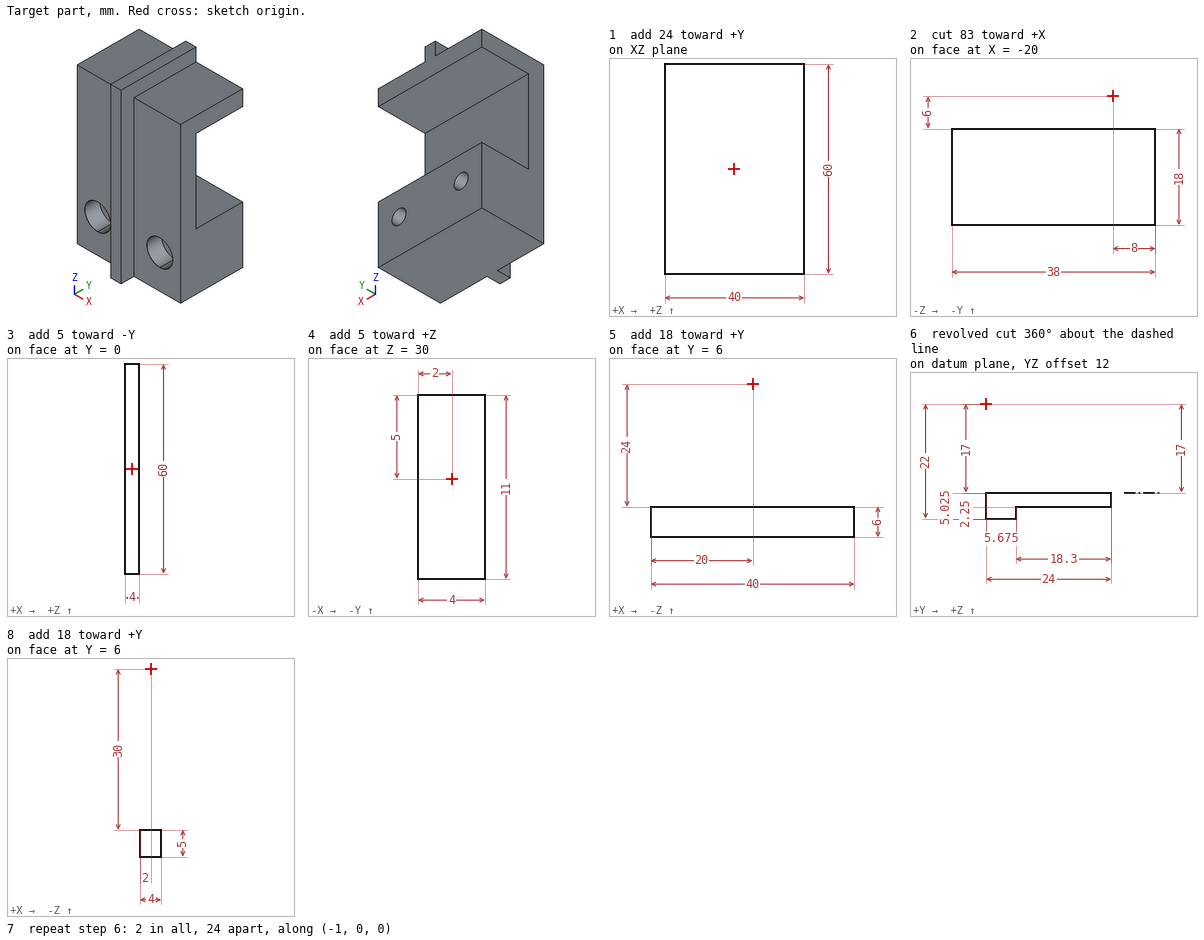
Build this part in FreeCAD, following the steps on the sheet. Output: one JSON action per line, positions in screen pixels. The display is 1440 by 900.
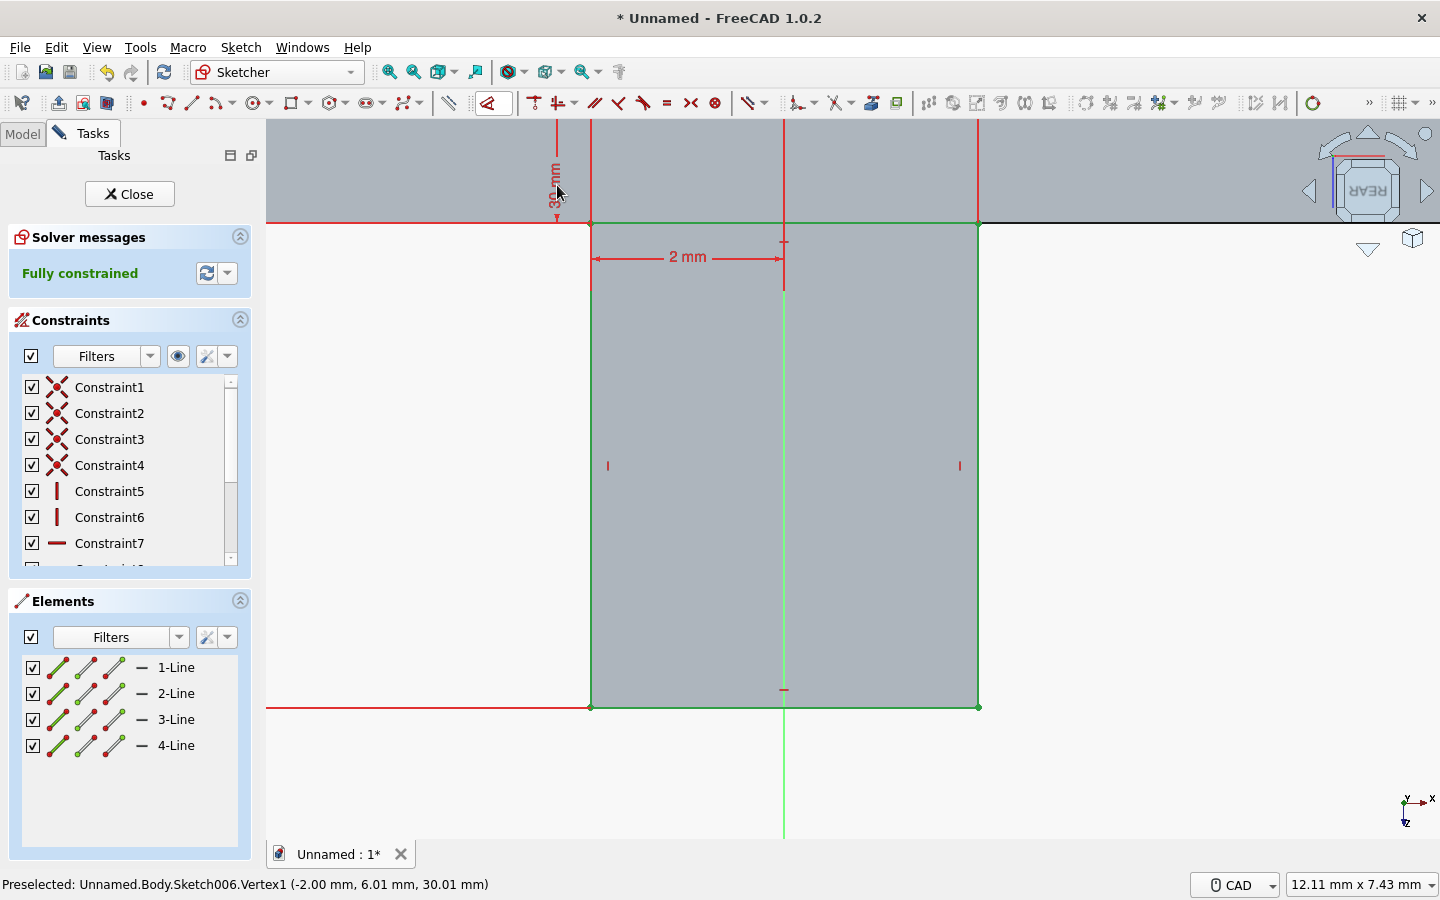
{"action": "left_click", "coordinate": [130, 194]}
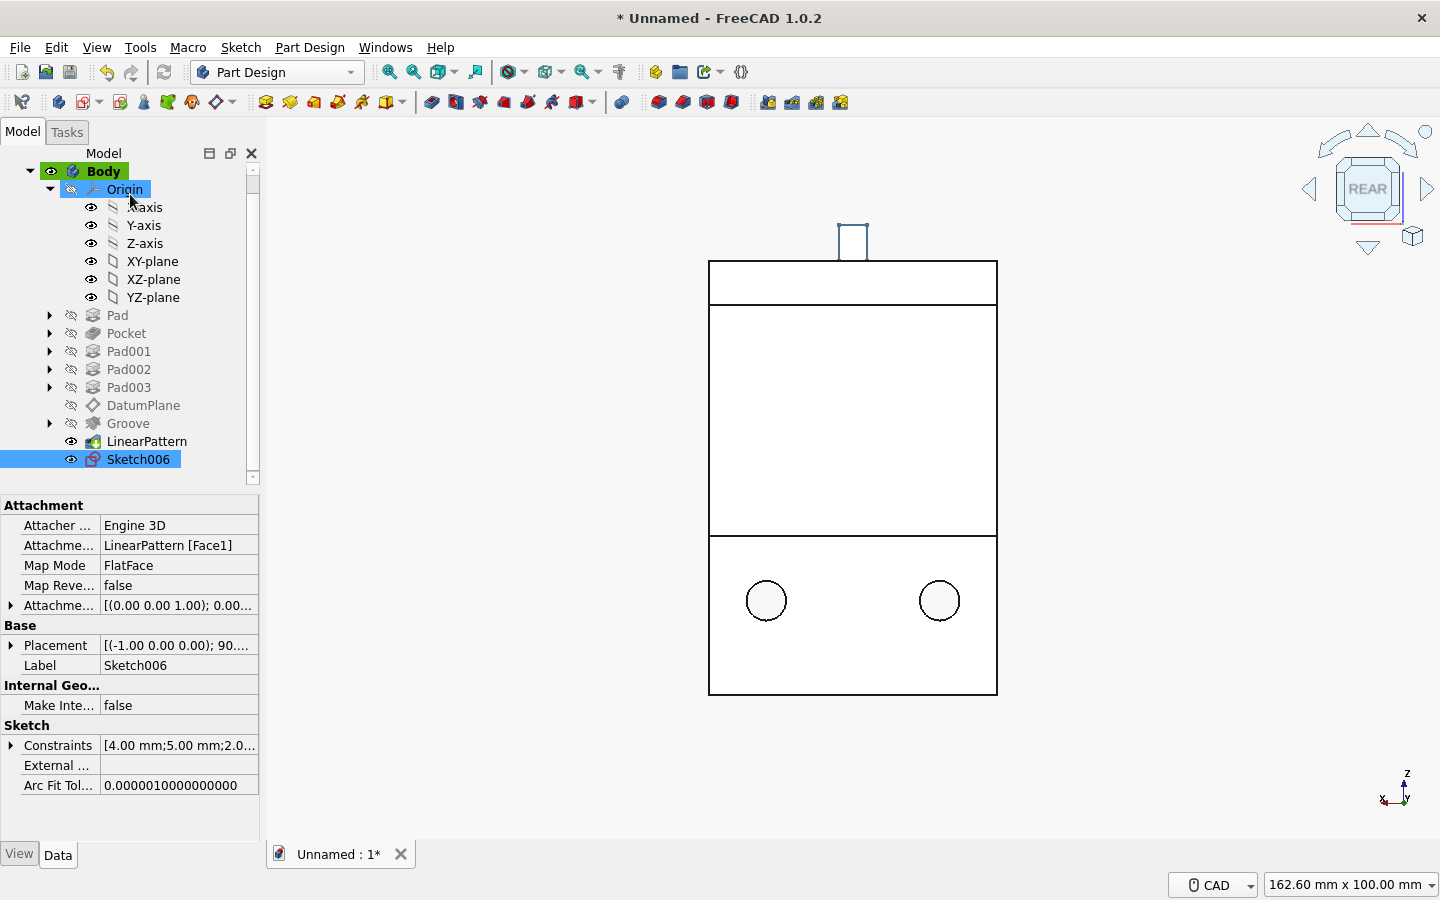
{"action": "left_click", "coordinate": [266, 102]}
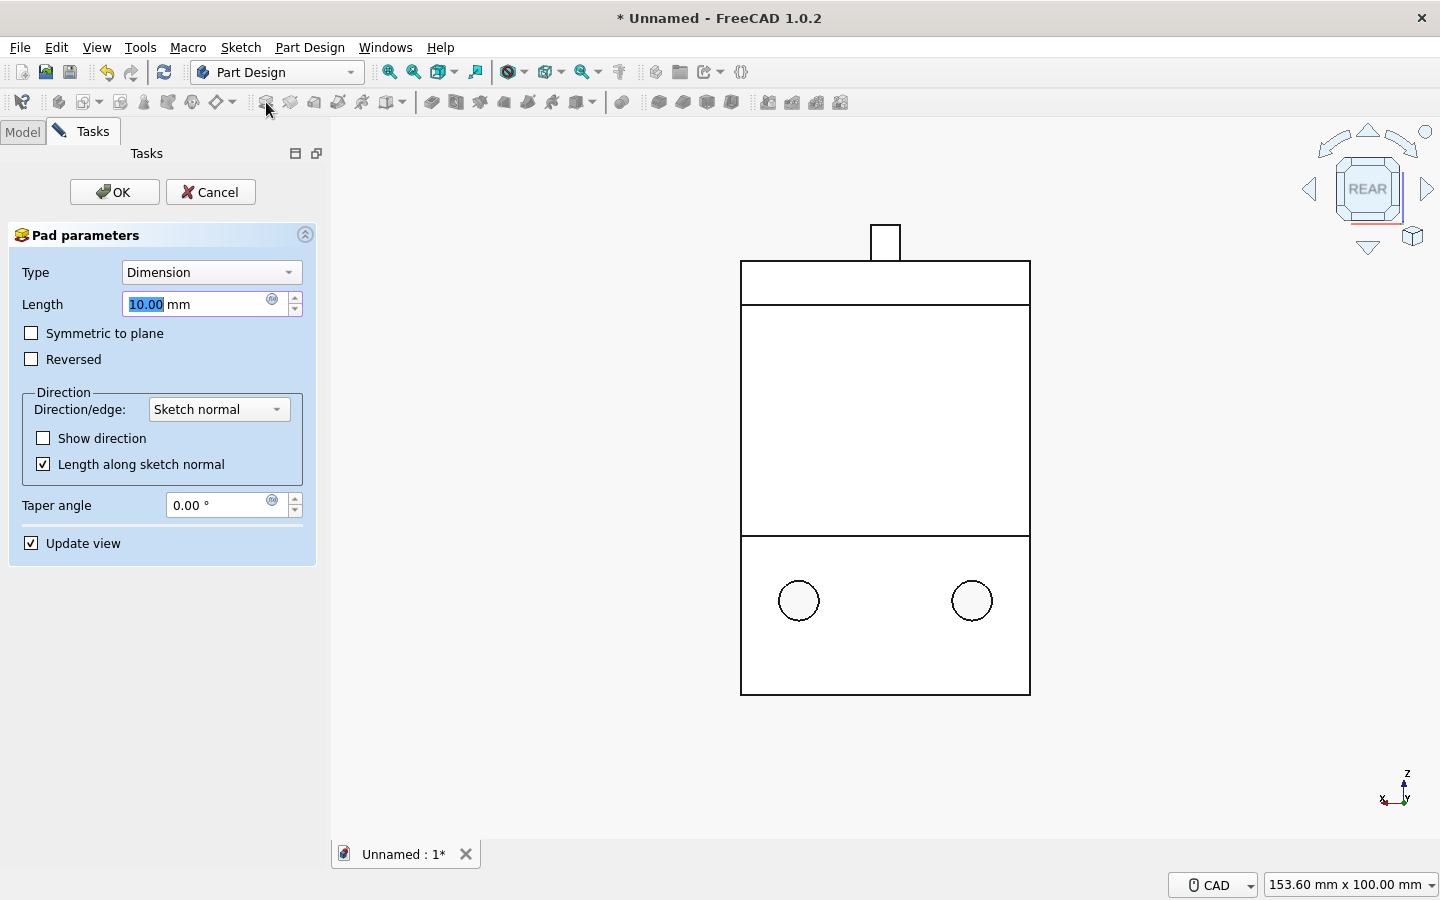
{"action": "type", "text": "18"}
{"action": "key", "text": "Tab"}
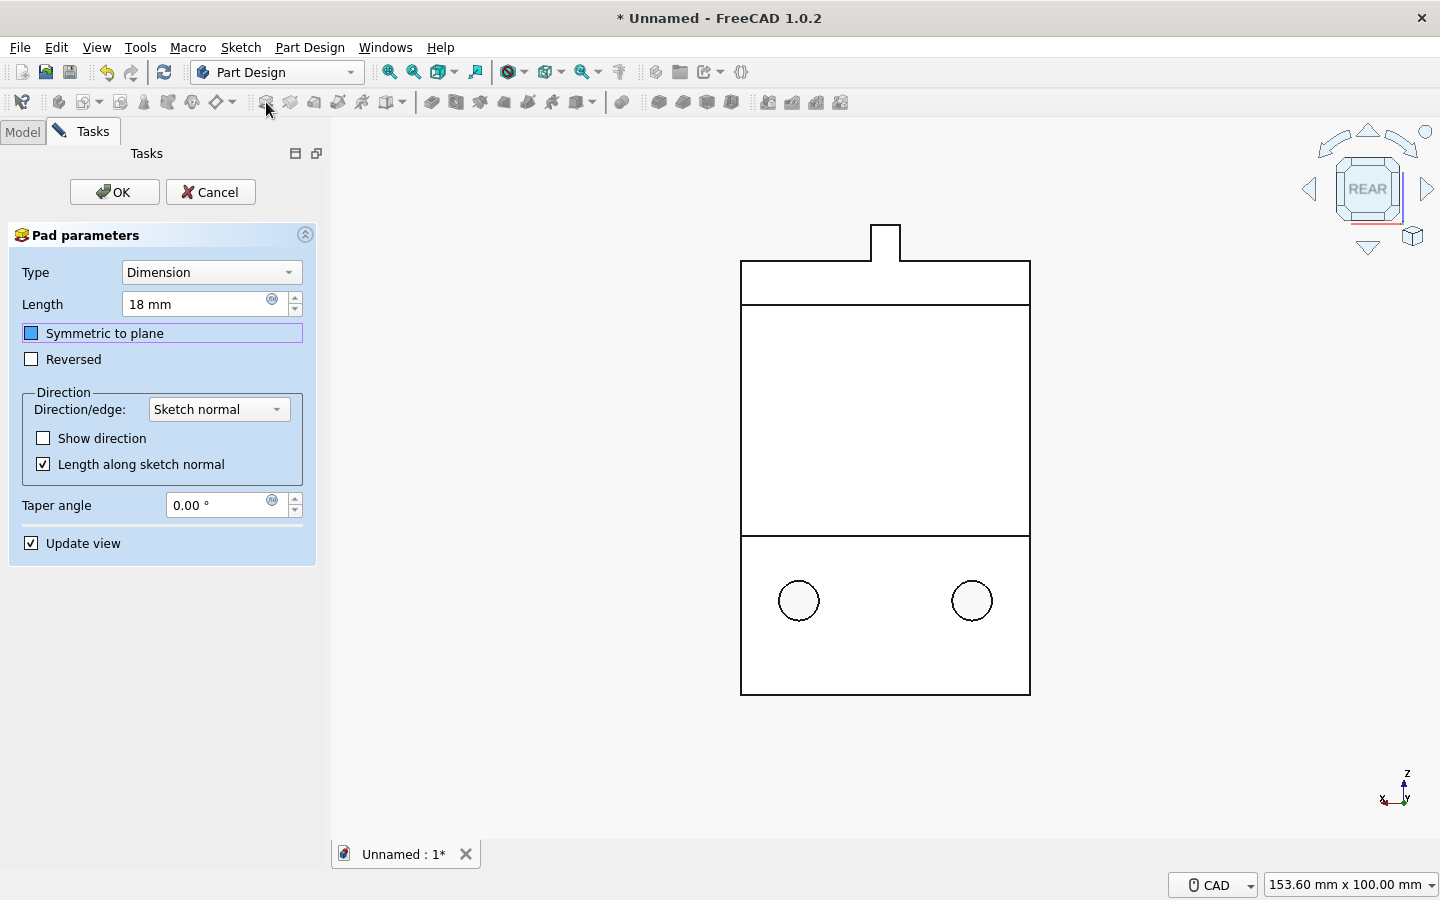
{"action": "left_click", "coordinate": [115, 192]}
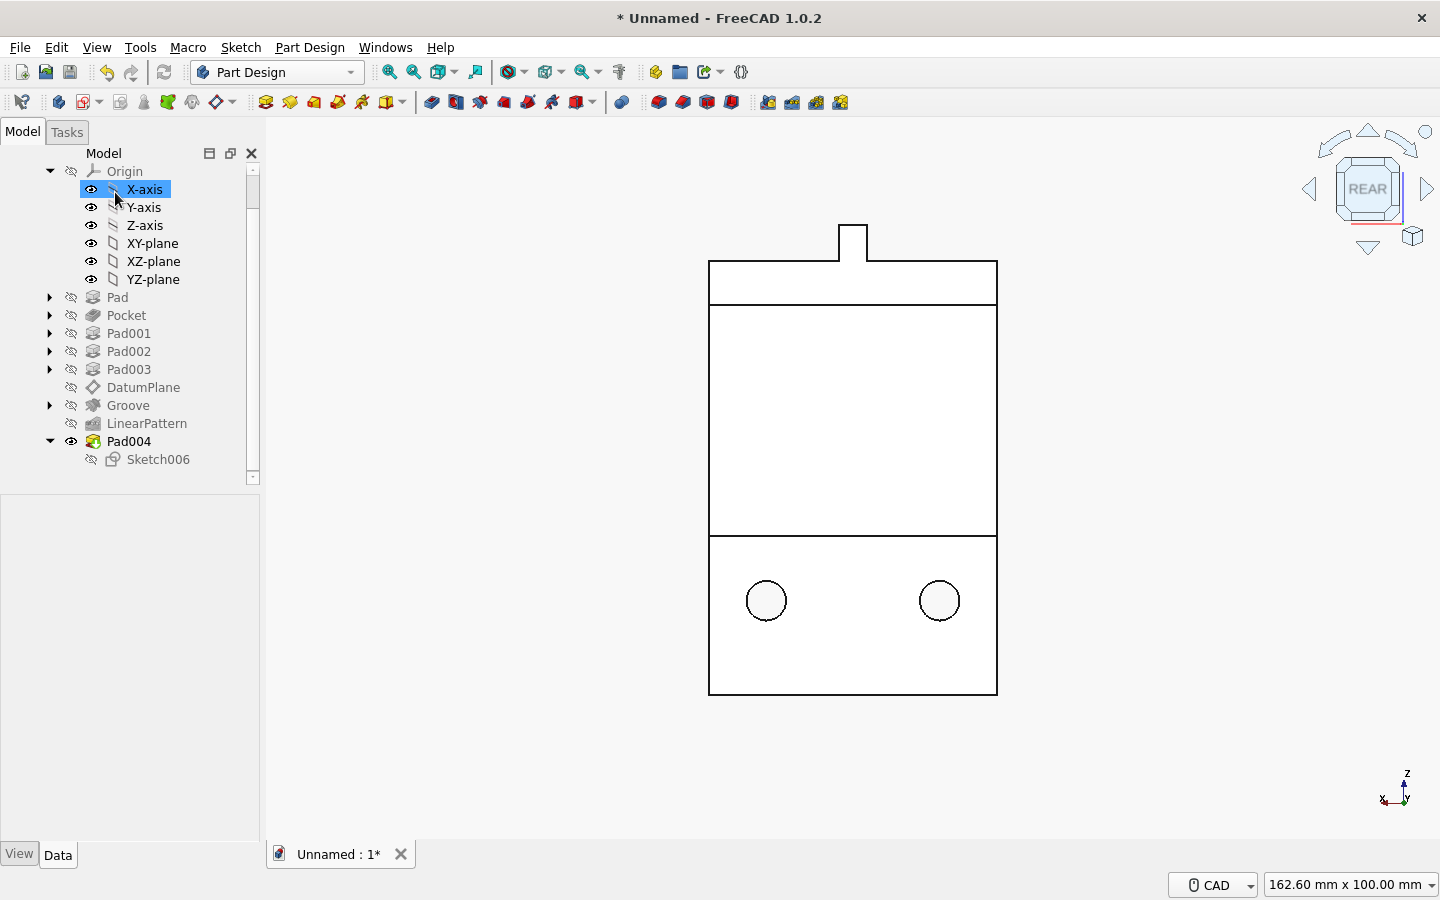
{"action": "key", "text": "0"}